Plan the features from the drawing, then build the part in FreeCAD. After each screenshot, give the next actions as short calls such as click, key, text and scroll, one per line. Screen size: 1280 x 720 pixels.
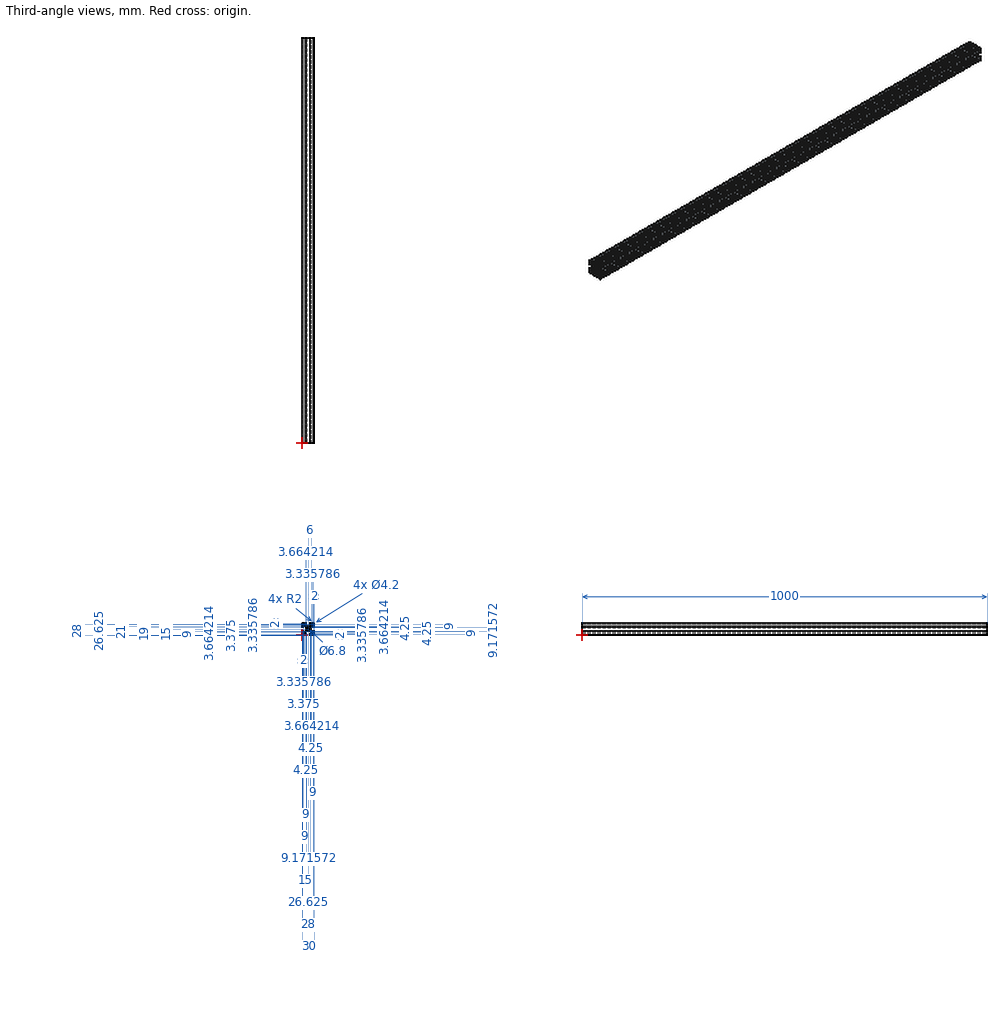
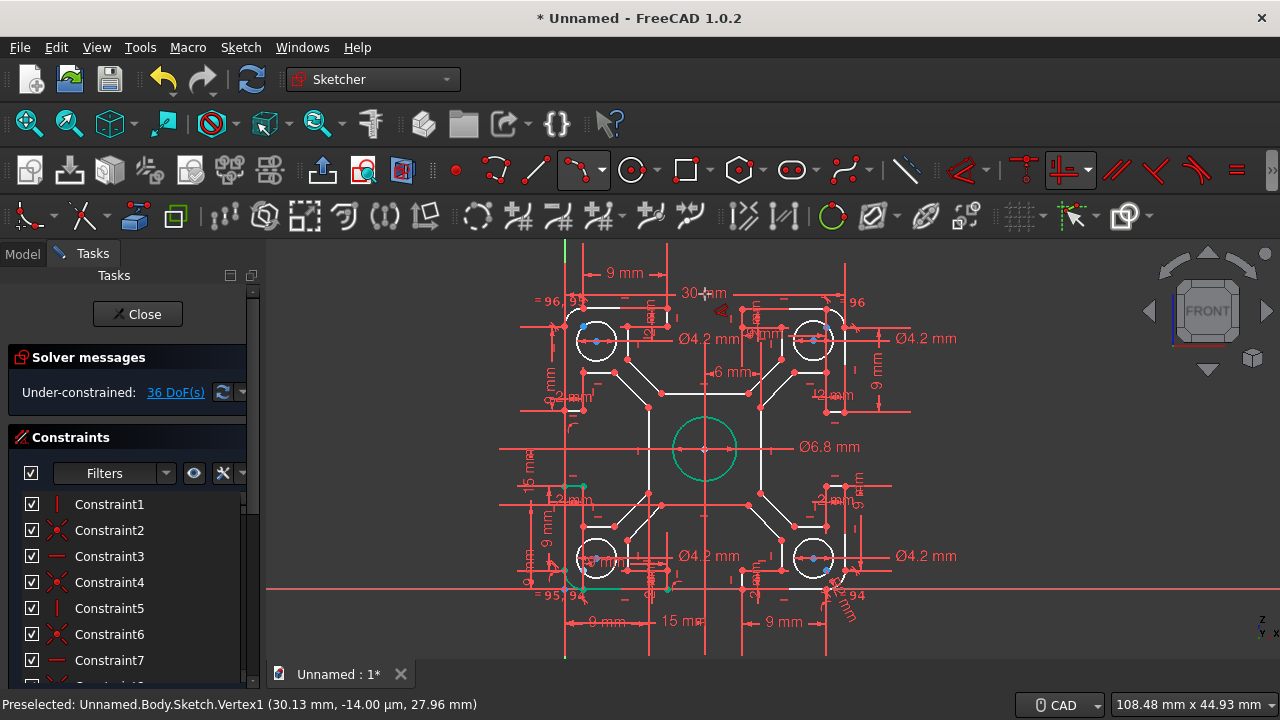
click(845, 328)
click(879, 459)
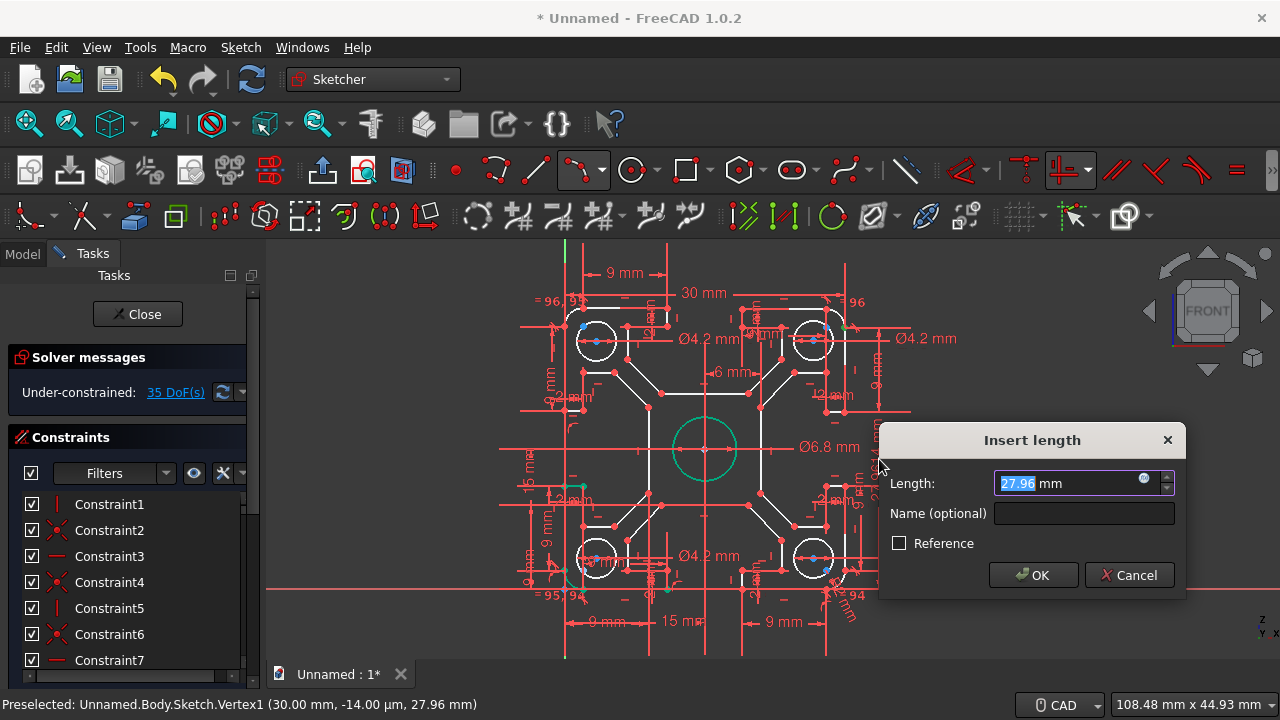
text(28)
key(Return)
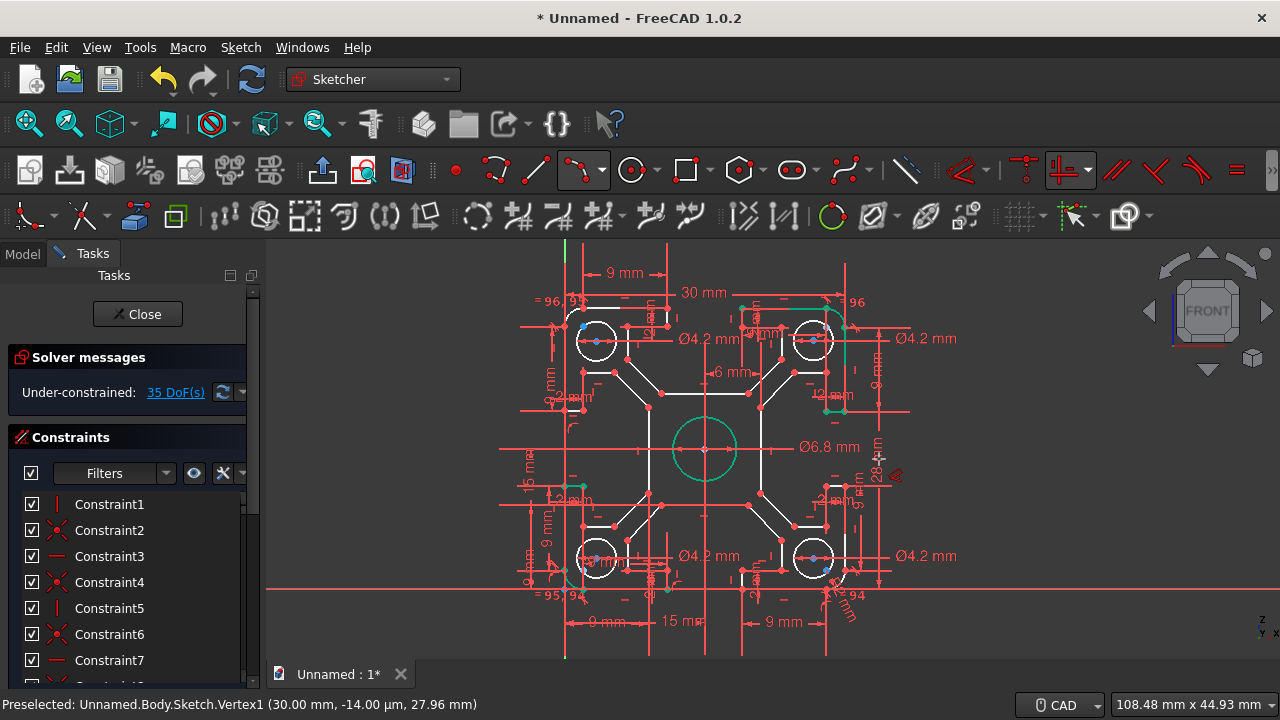
click(826, 527)
click(635, 469)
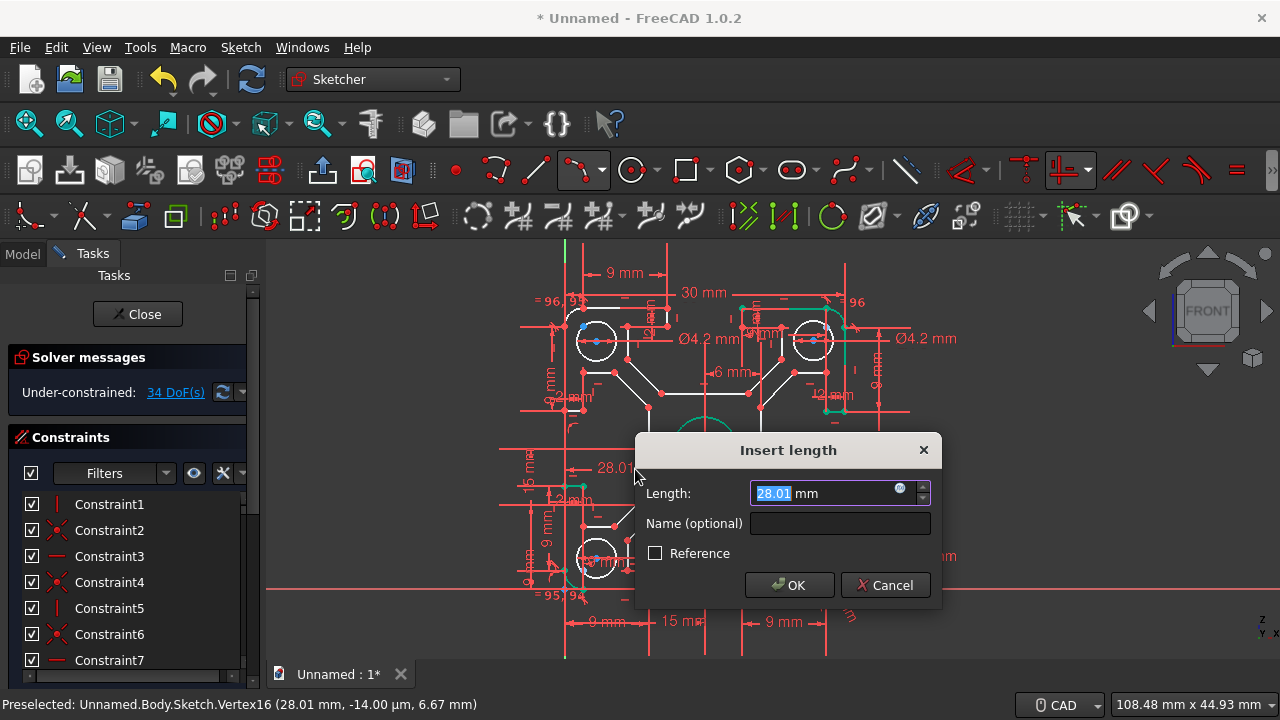
text(28)
key(Return)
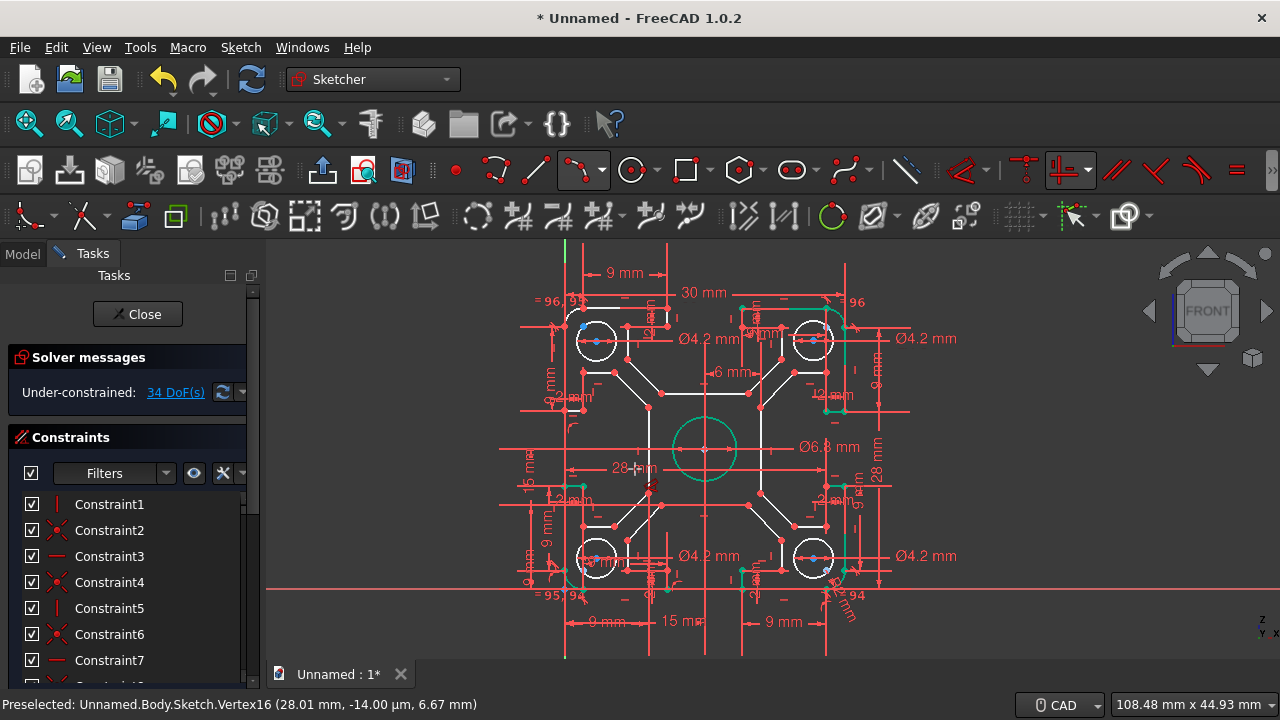
click(583, 411)
click(531, 438)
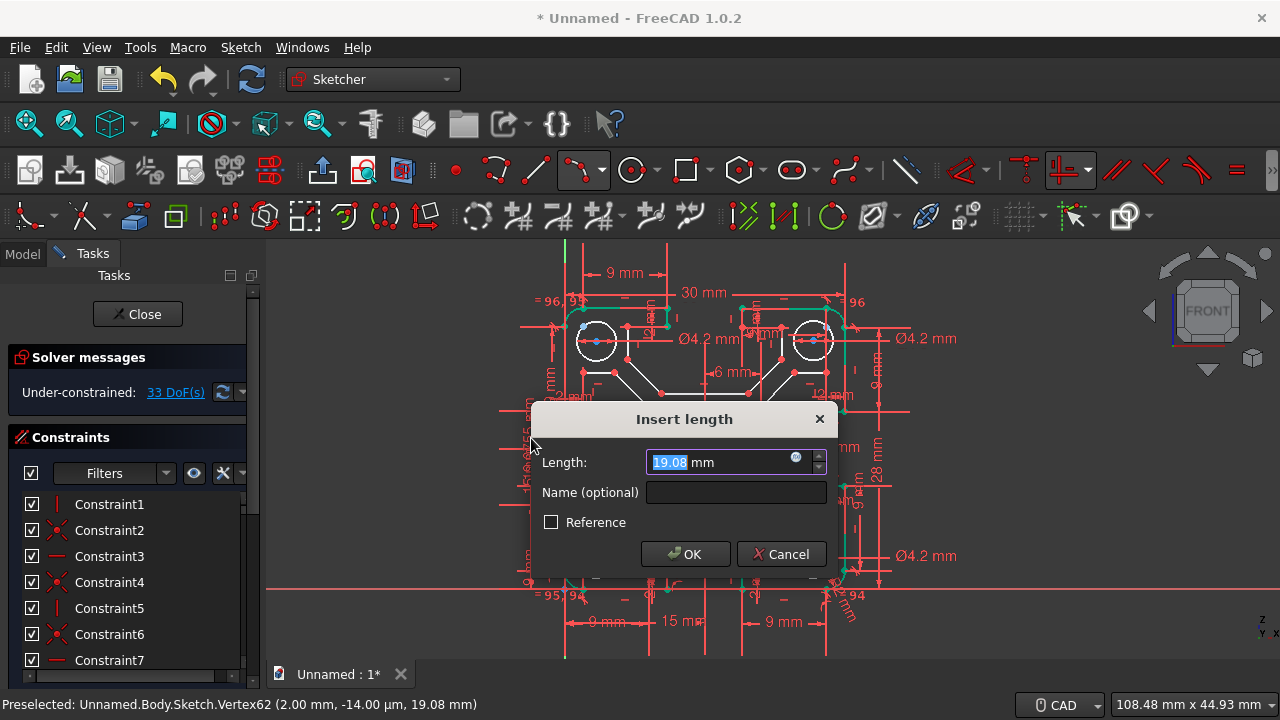
text(19)
key(Return)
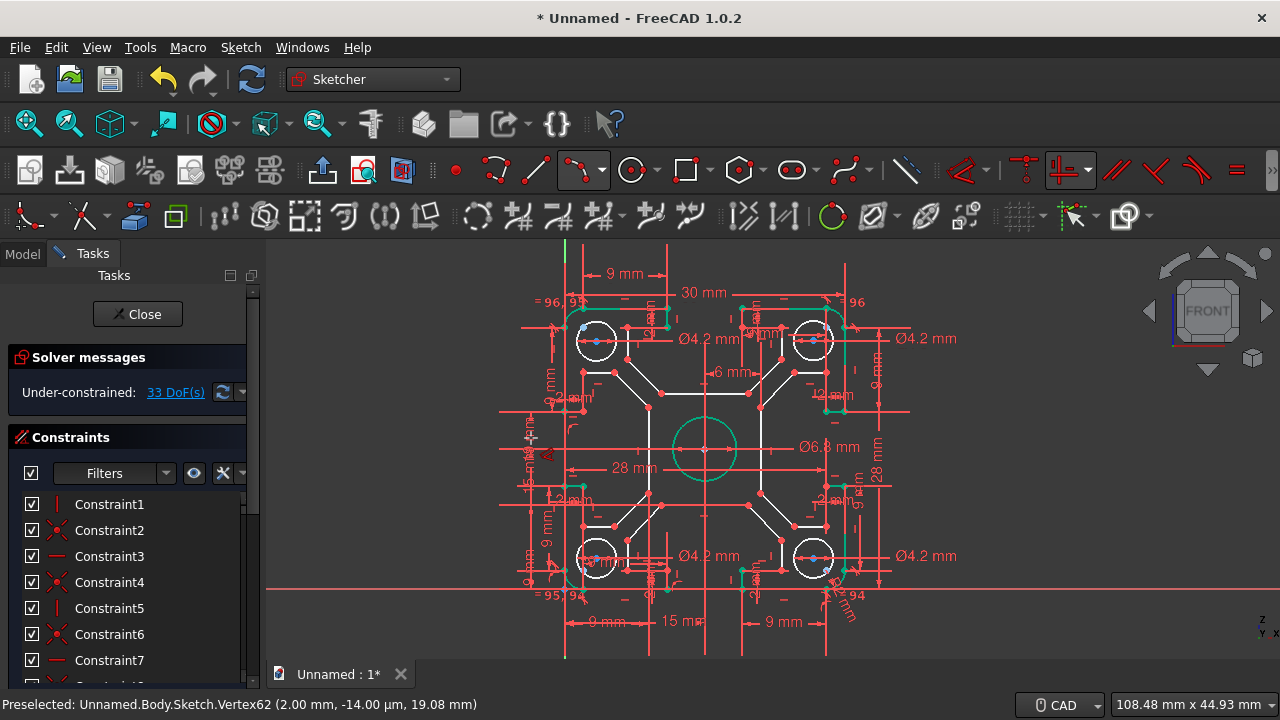
click(661, 394)
click(695, 446)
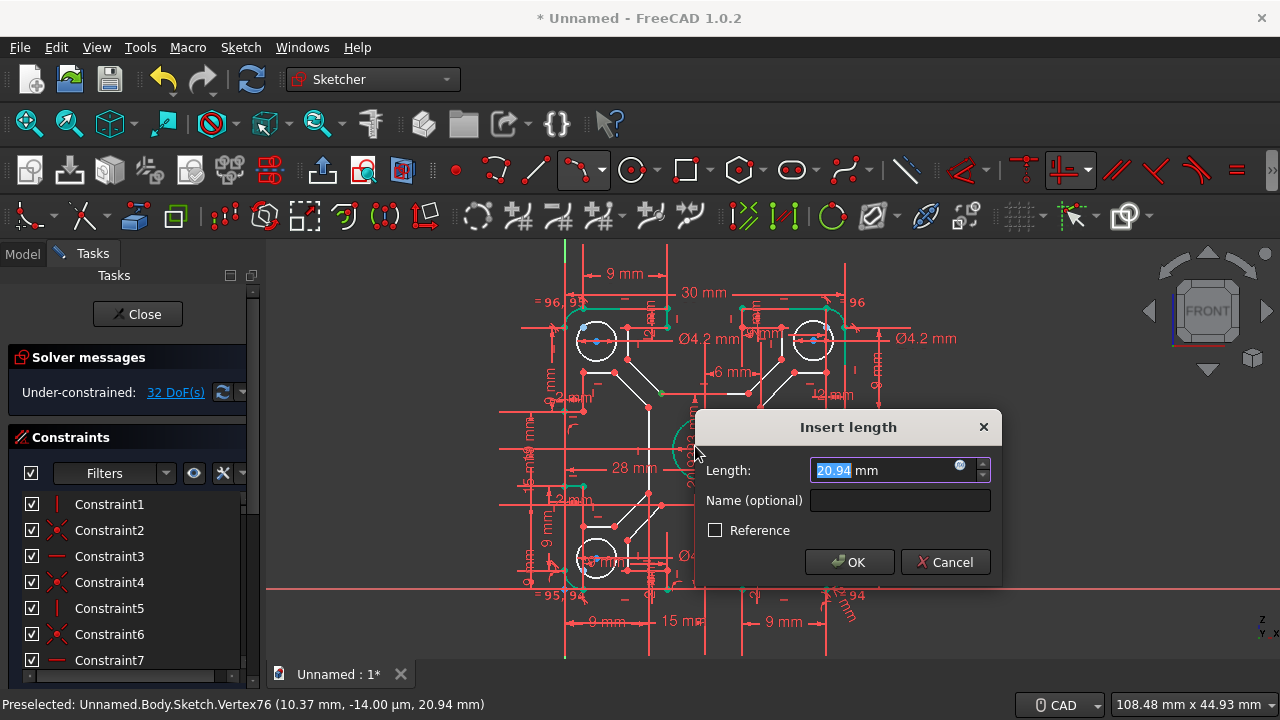
text(21)
key(Return)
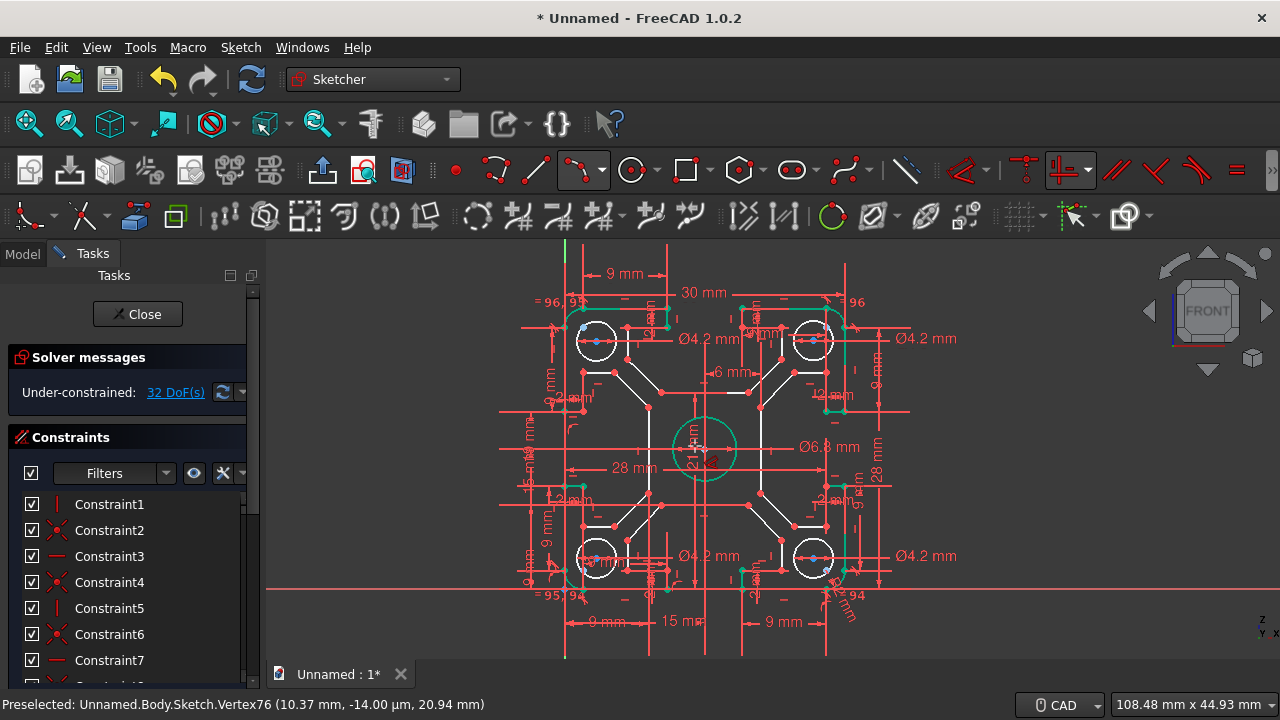
click(826, 400)
click(908, 392)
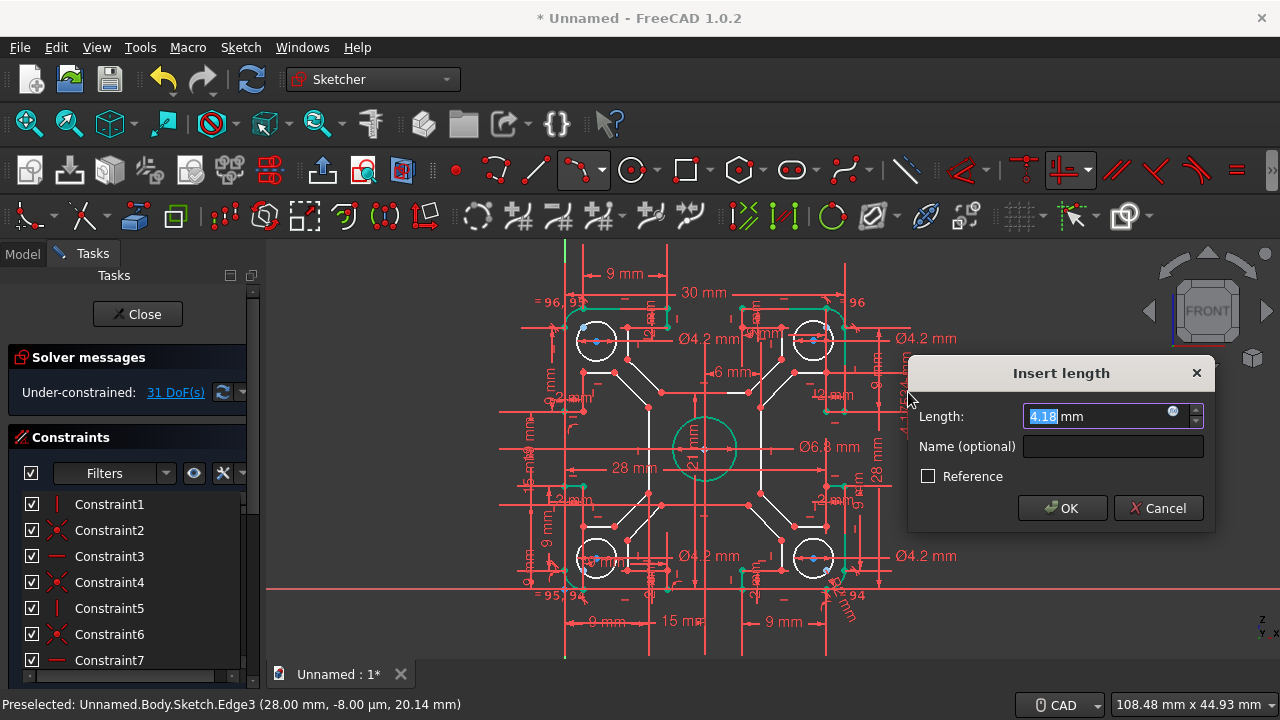
text(4.25)
key(Return)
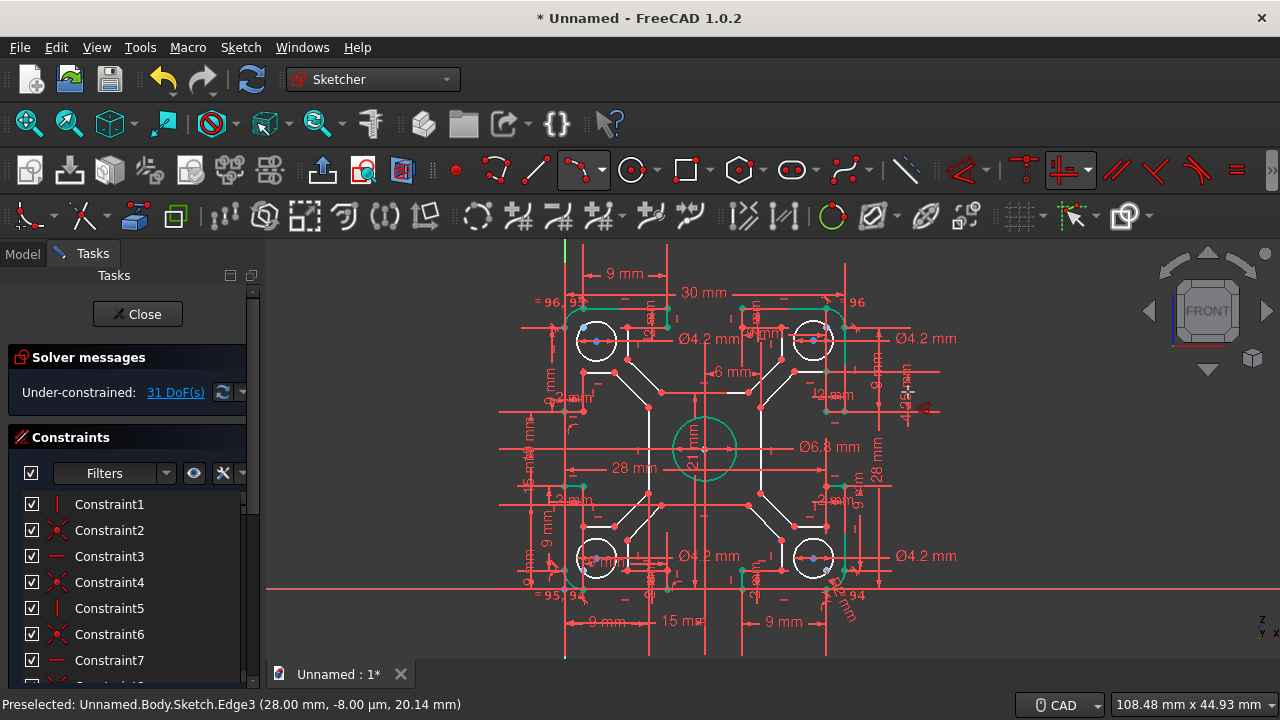
click(826, 515)
click(908, 516)